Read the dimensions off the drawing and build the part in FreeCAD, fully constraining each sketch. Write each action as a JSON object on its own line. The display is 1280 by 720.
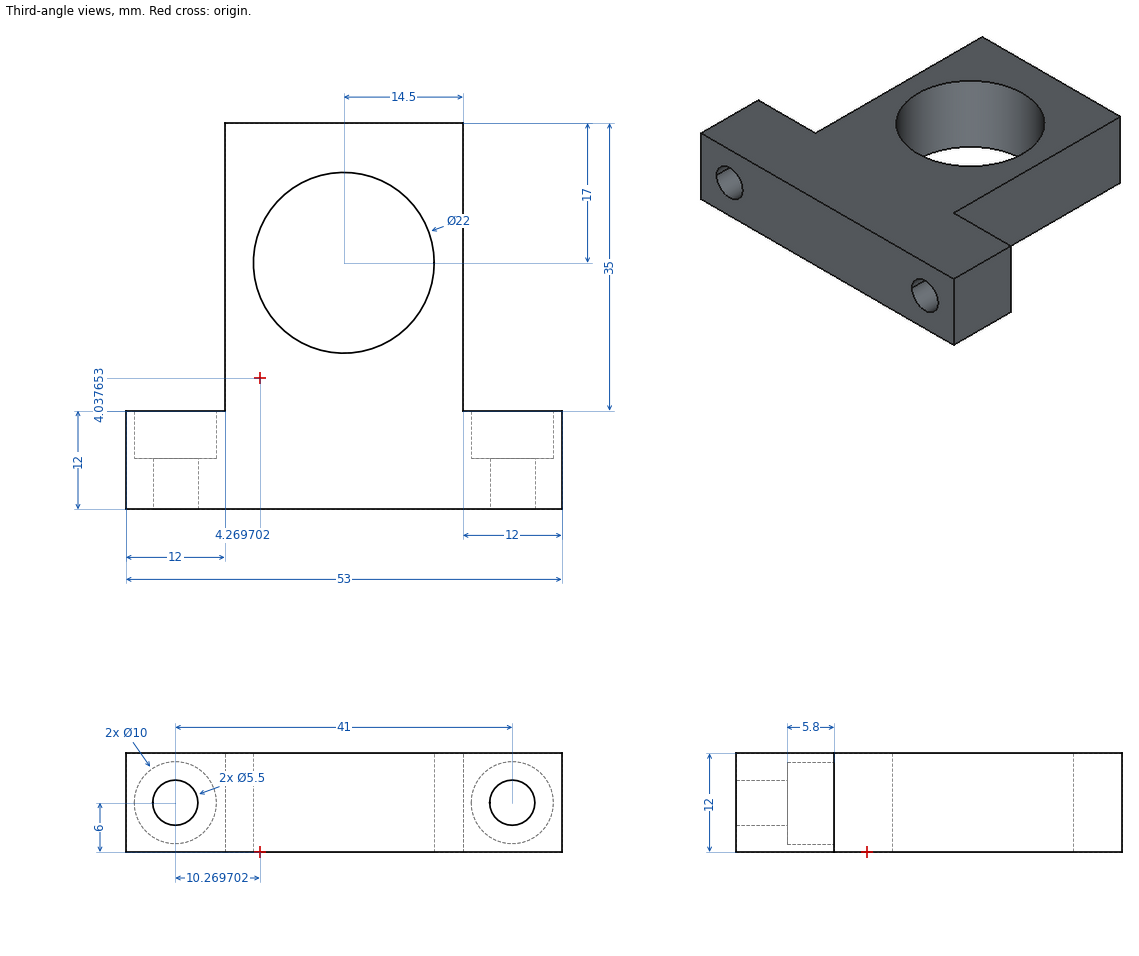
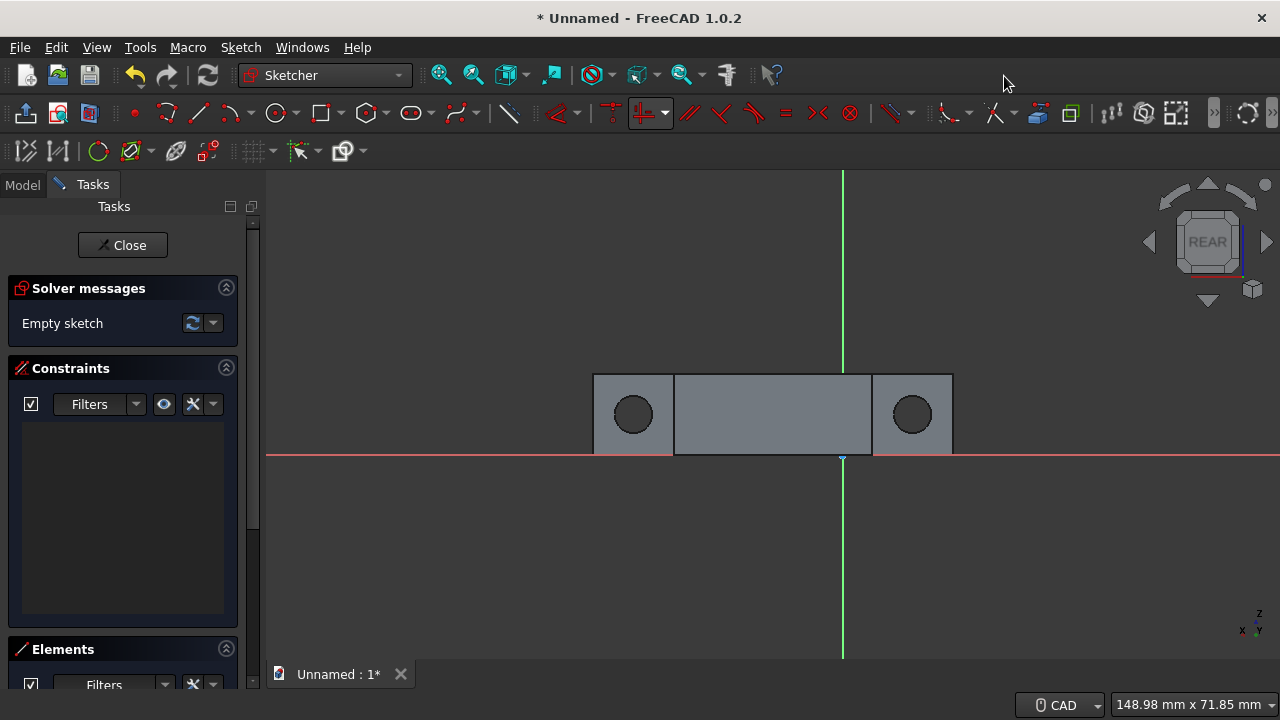
{"action": "scroll", "coordinate": [856, 422], "scroll_direction": "up", "scroll_amount": 3}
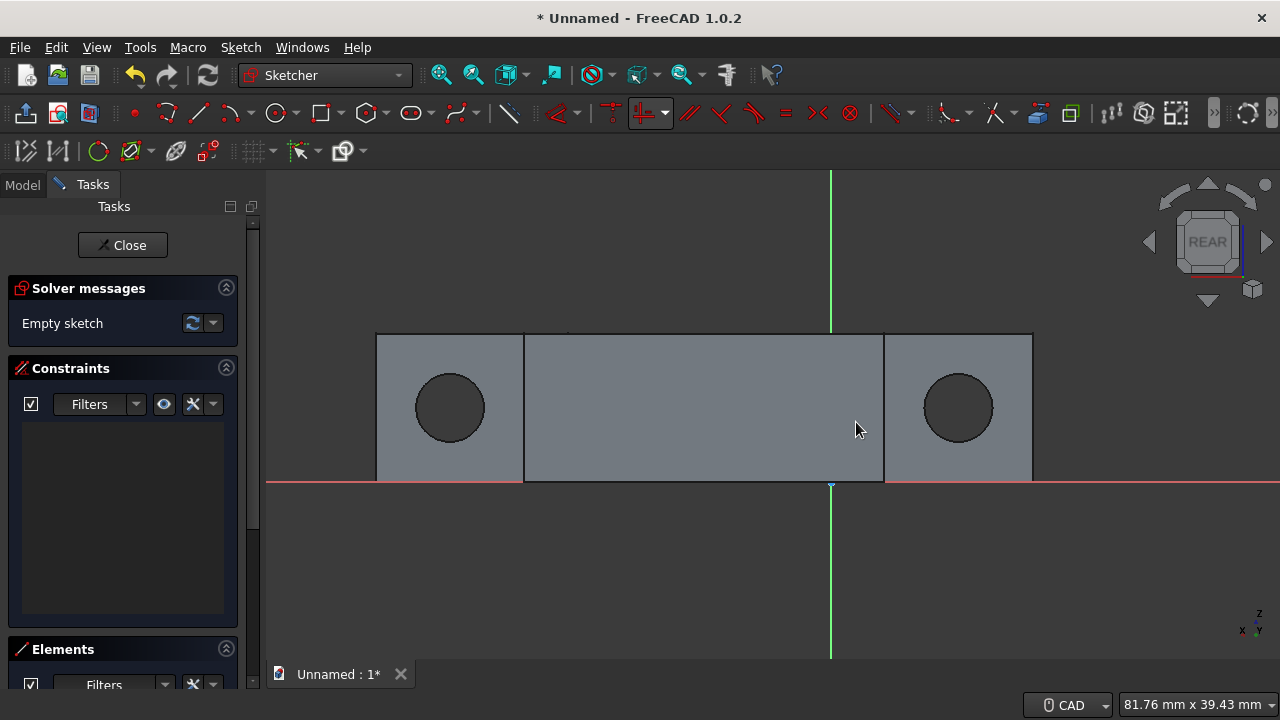
{"action": "left_click", "coordinate": [276, 114]}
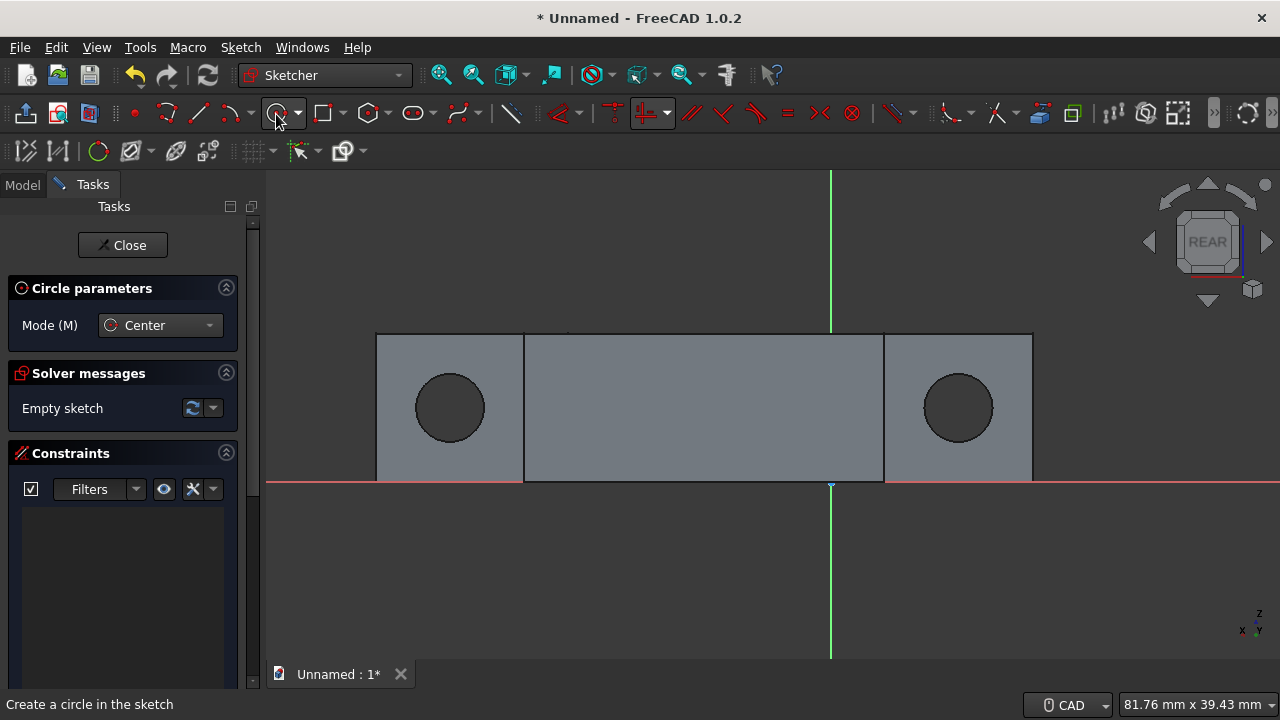
{"action": "left_click", "coordinate": [959, 408]}
{"action": "mouse_move", "coordinate": [1002, 364]}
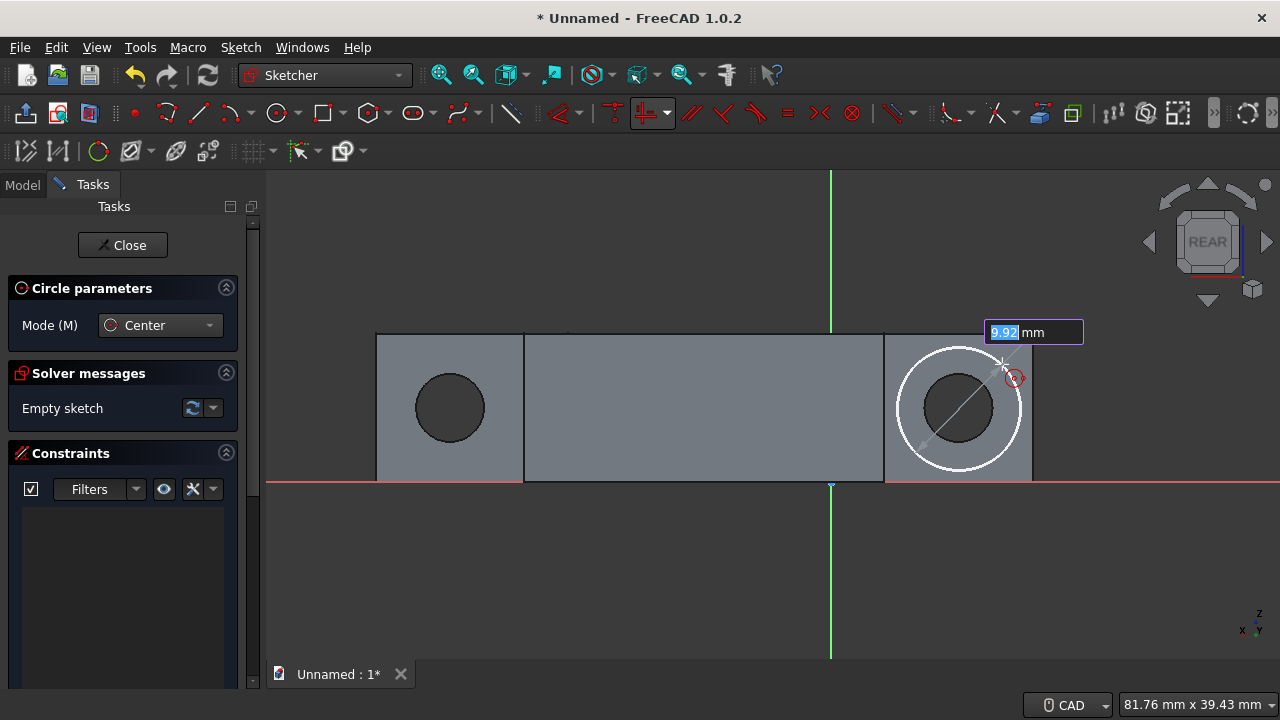
{"action": "type", "text": "10"}
{"action": "key", "text": "Return"}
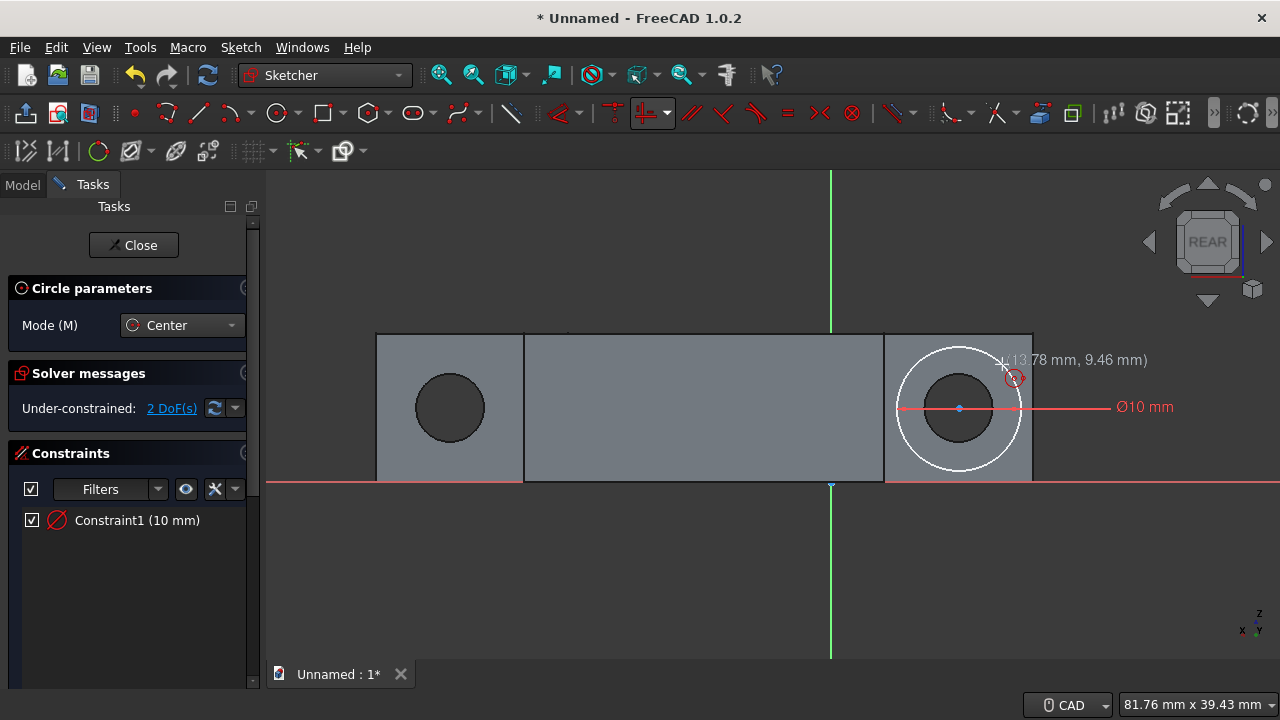
{"action": "left_click", "coordinate": [450, 408]}
{"action": "mouse_move", "coordinate": [494, 364]}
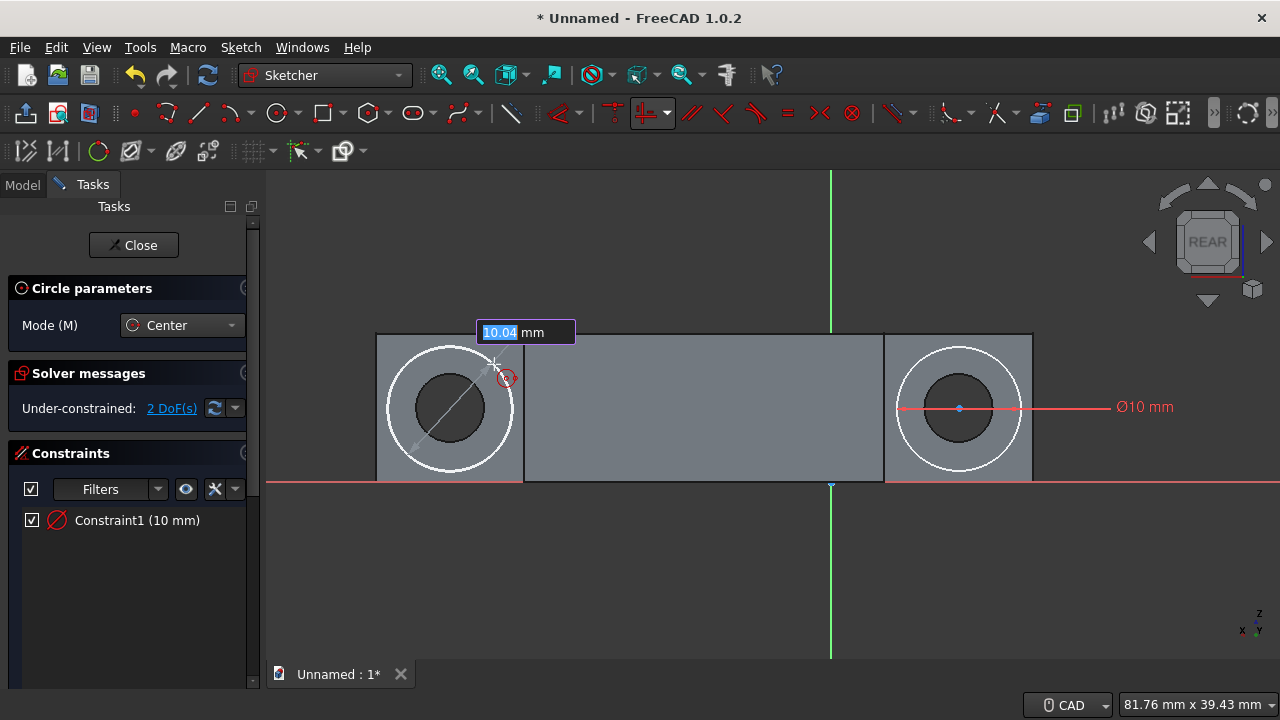
{"action": "type", "text": "10"}
{"action": "key", "text": "Return"}
{"action": "key", "text": "Escape"}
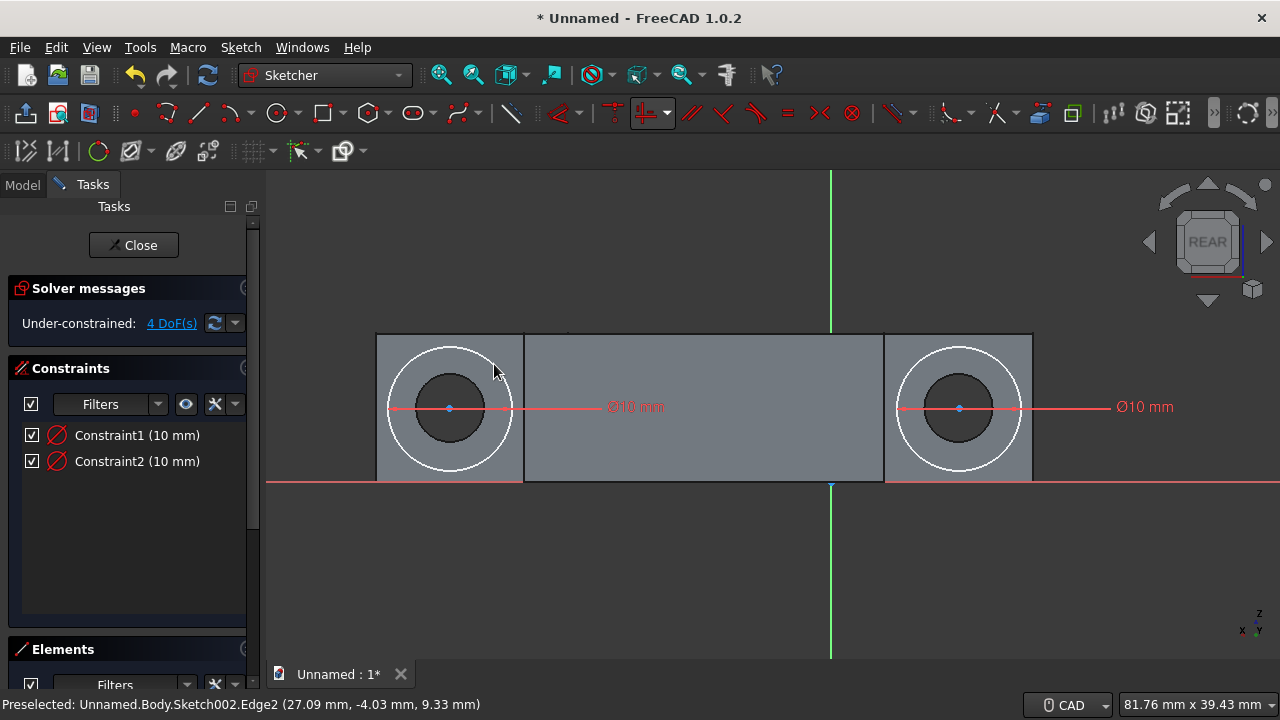
{"action": "left_click", "coordinate": [558, 114]}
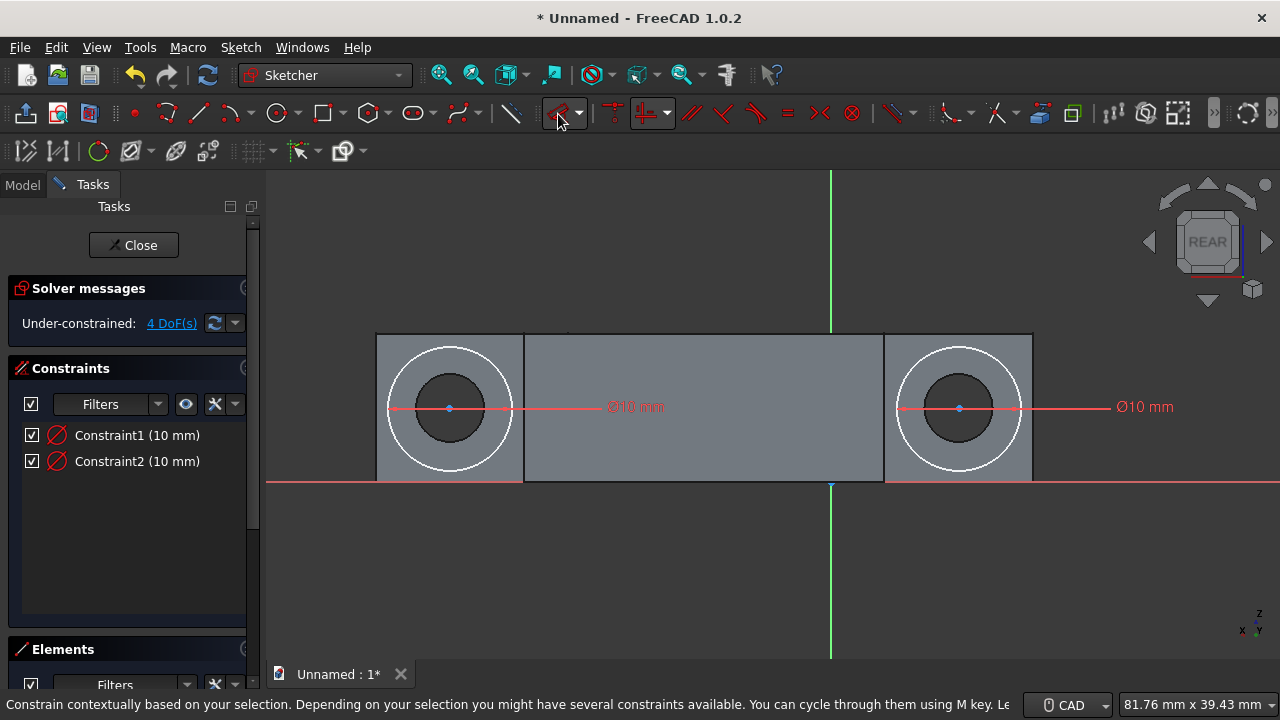
{"action": "left_click", "coordinate": [959, 409]}
{"action": "left_click", "coordinate": [993, 429]}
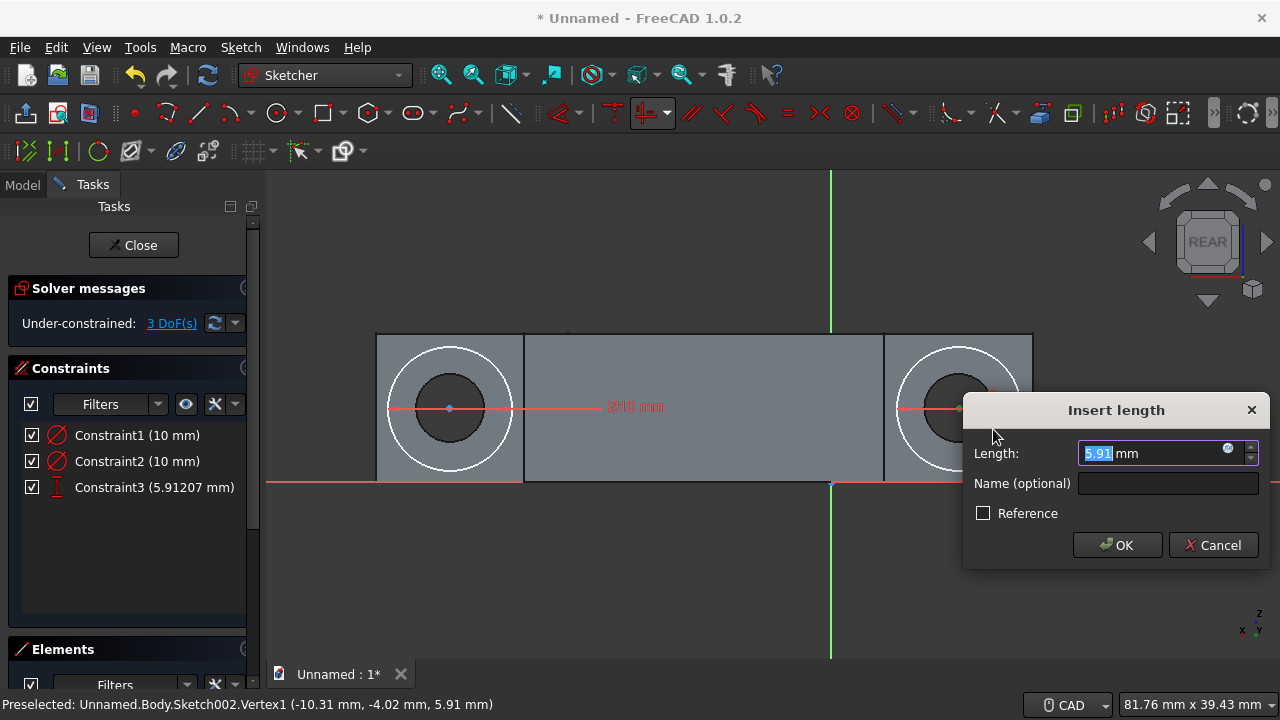
{"action": "type", "text": "6"}
{"action": "key", "text": "Return"}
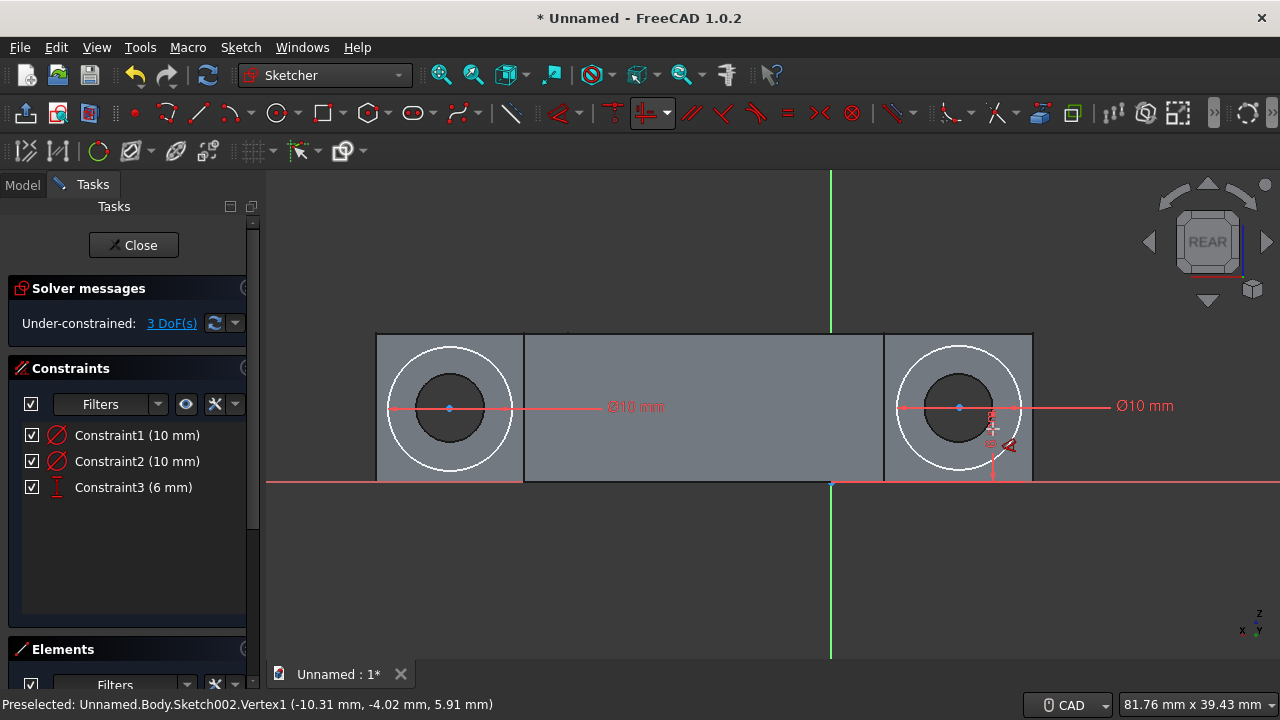
{"action": "left_click", "coordinate": [450, 409]}
{"action": "left_click", "coordinate": [416, 429]}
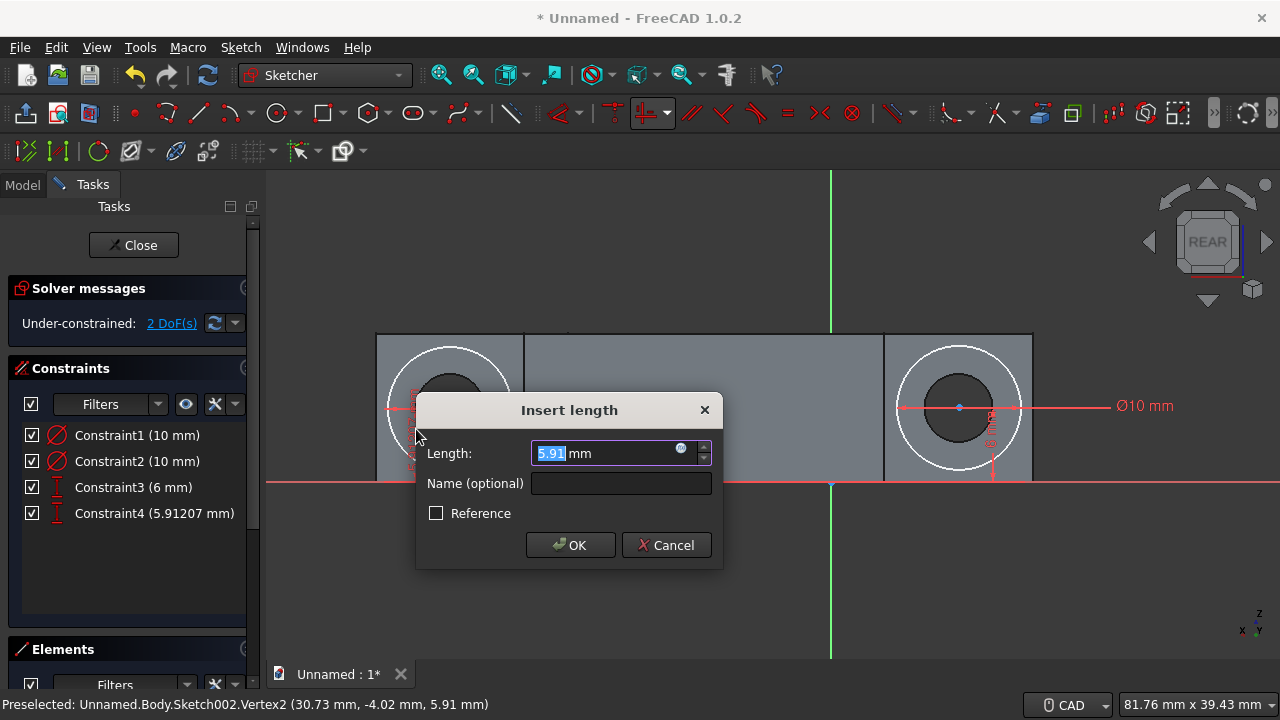
{"action": "type", "text": "6"}
{"action": "key", "text": "Return"}